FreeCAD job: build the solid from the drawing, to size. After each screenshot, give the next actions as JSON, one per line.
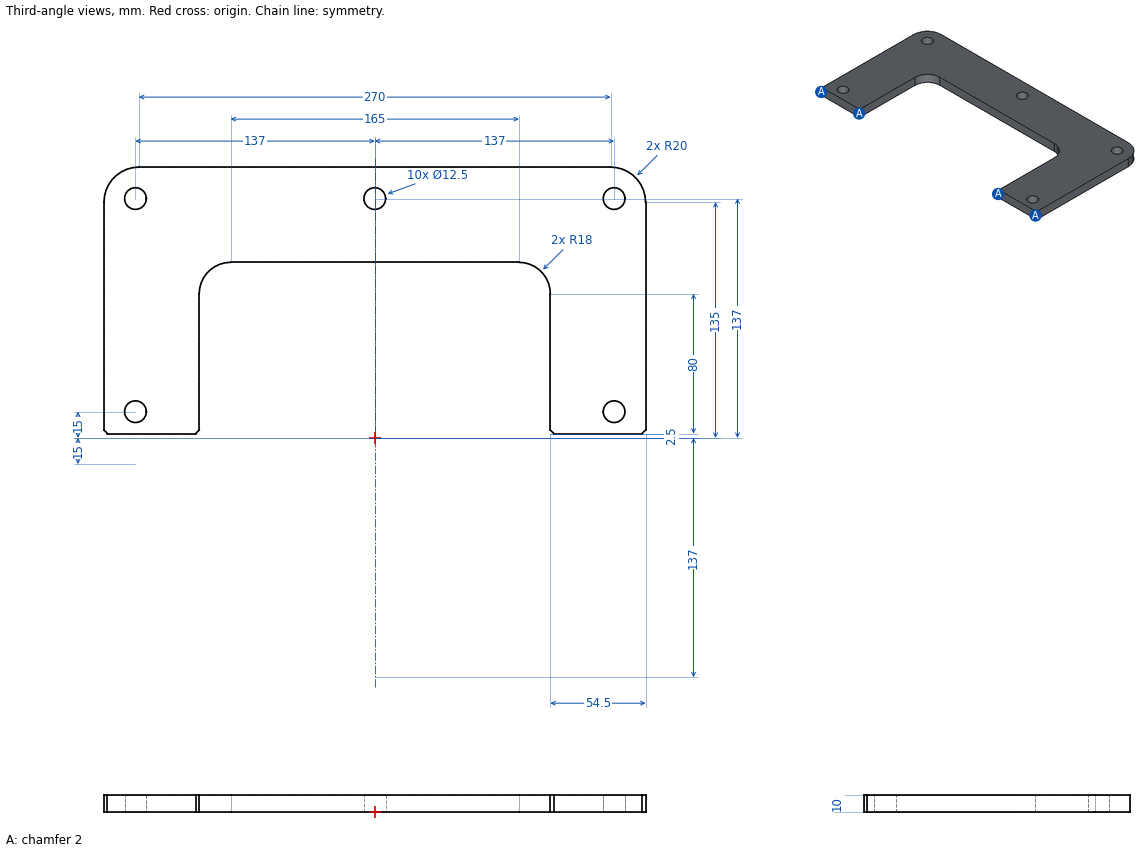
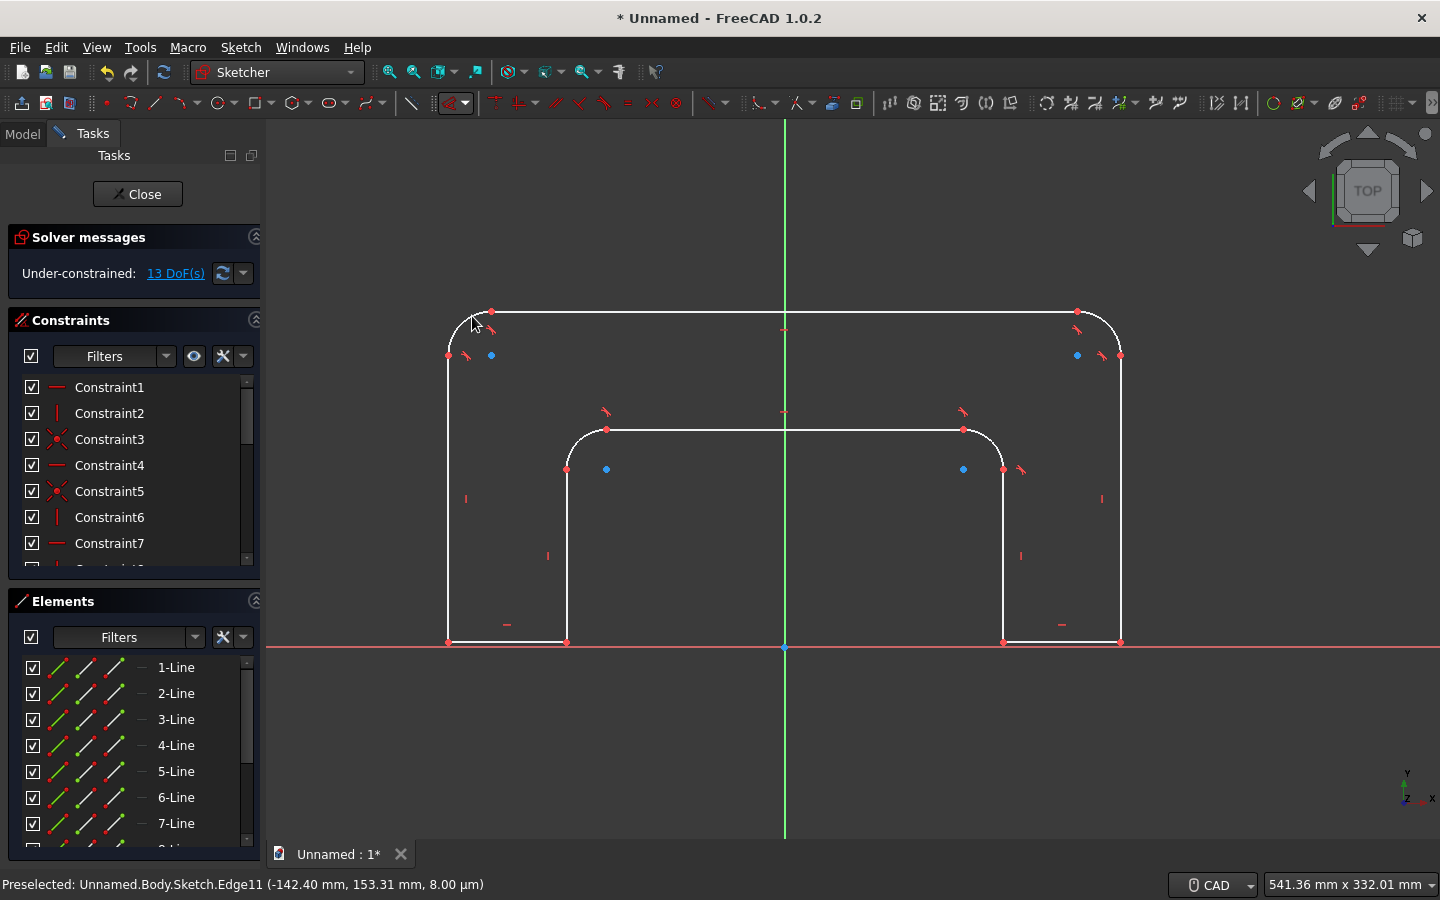
{"action": "left_click", "coordinate": [567, 590]}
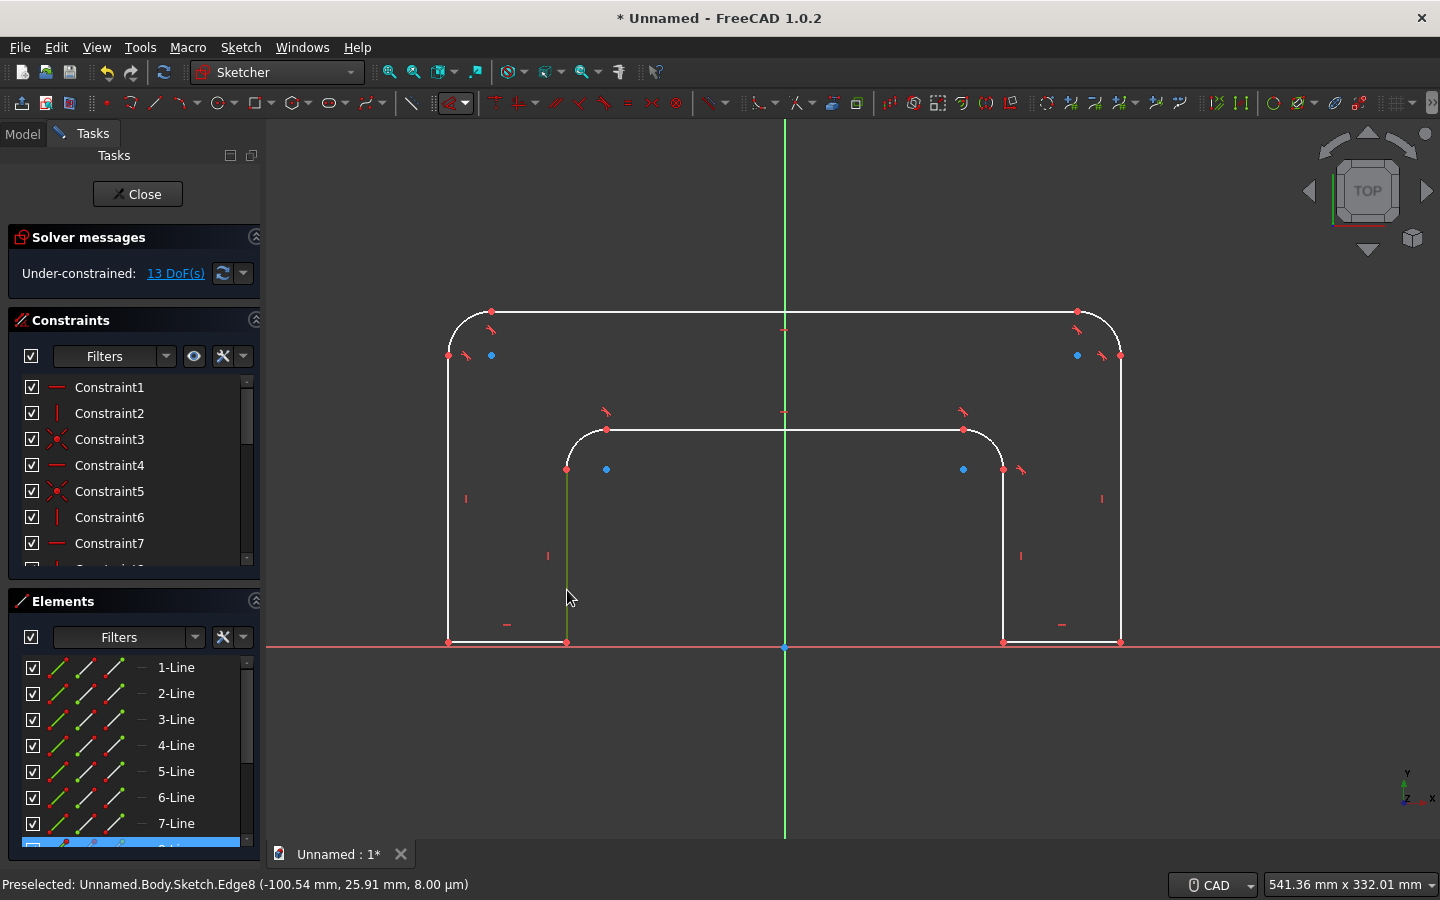
{"action": "left_click", "coordinate": [588, 434]}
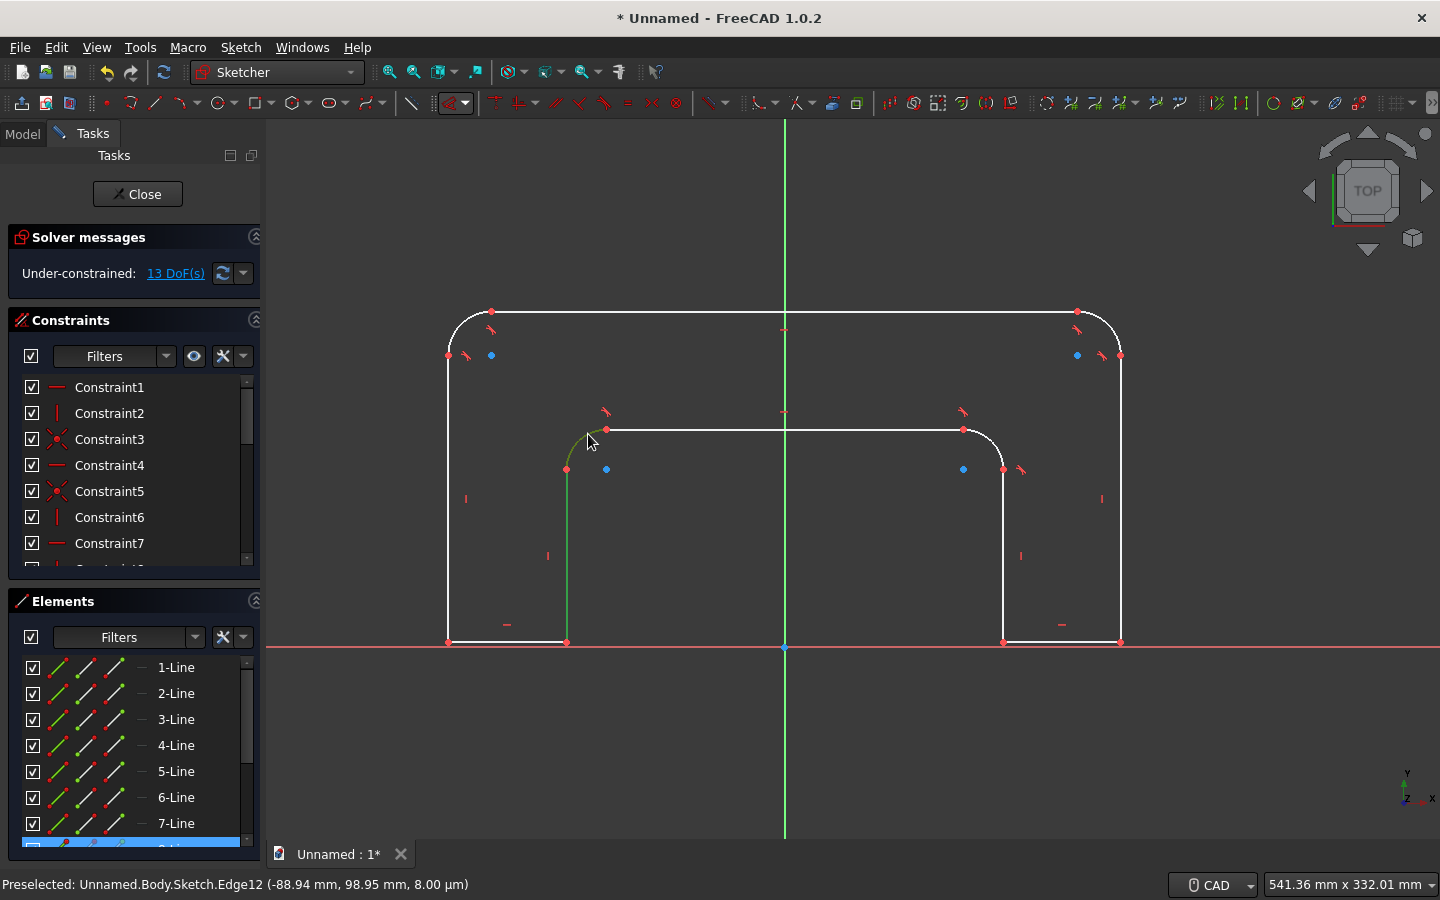
{"action": "key", "text": "t"}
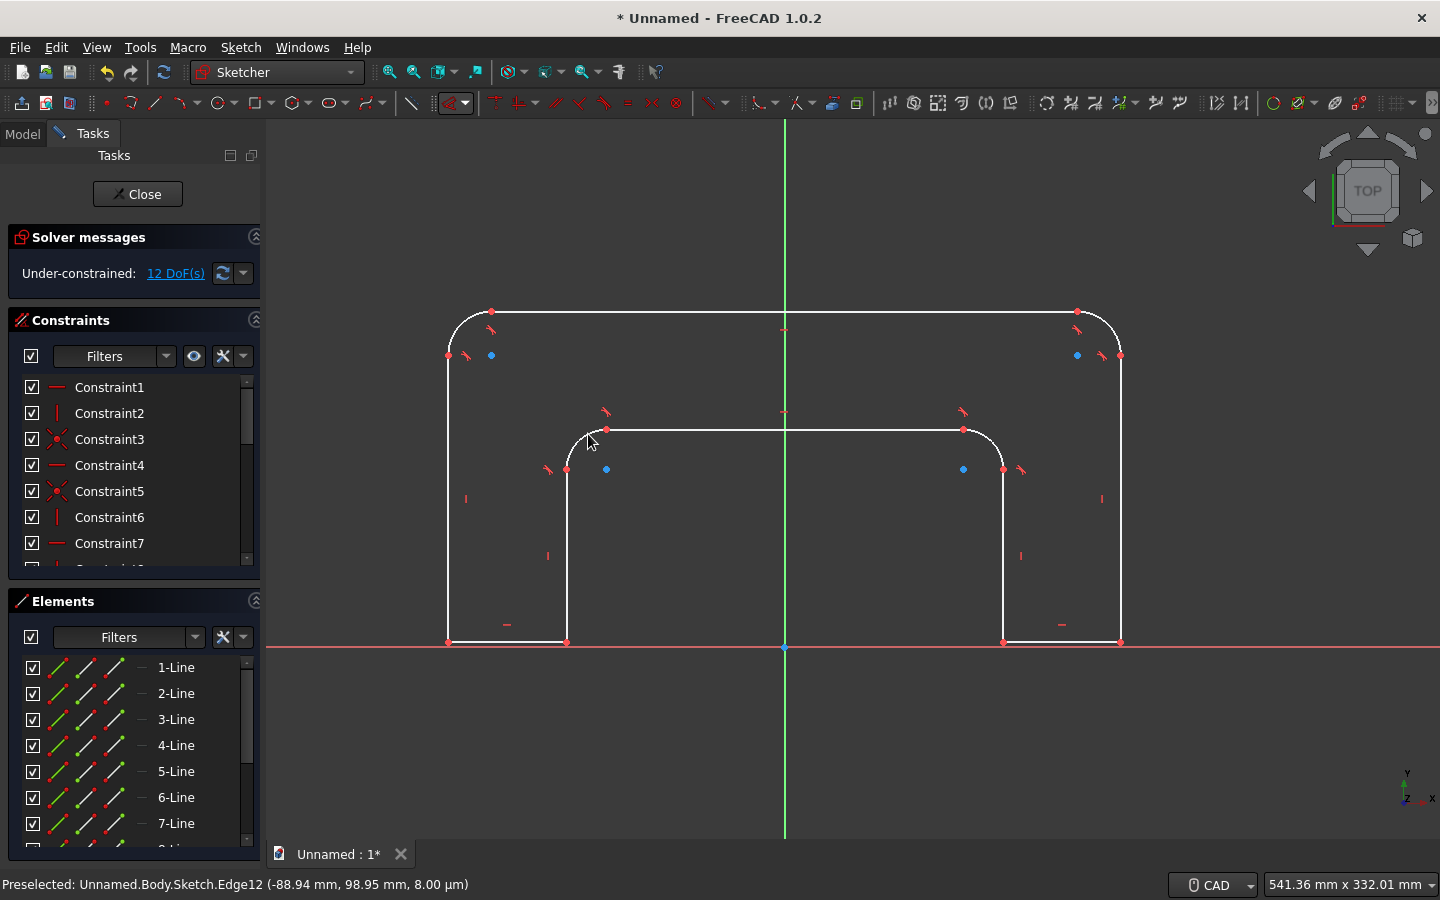
{"action": "left_click", "coordinate": [1116, 336]}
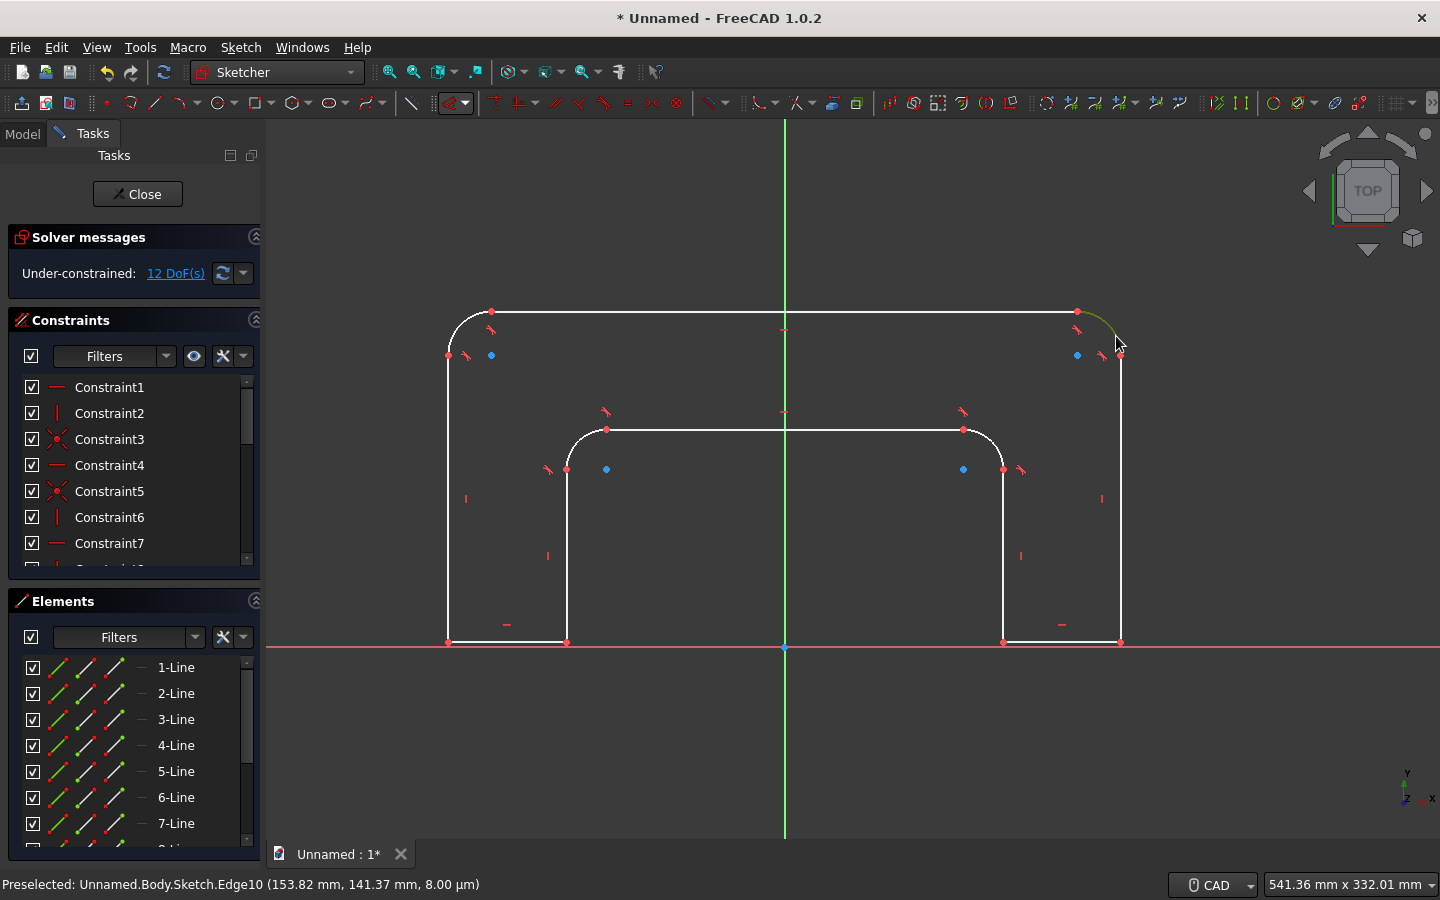
{"action": "left_click", "coordinate": [472, 316]}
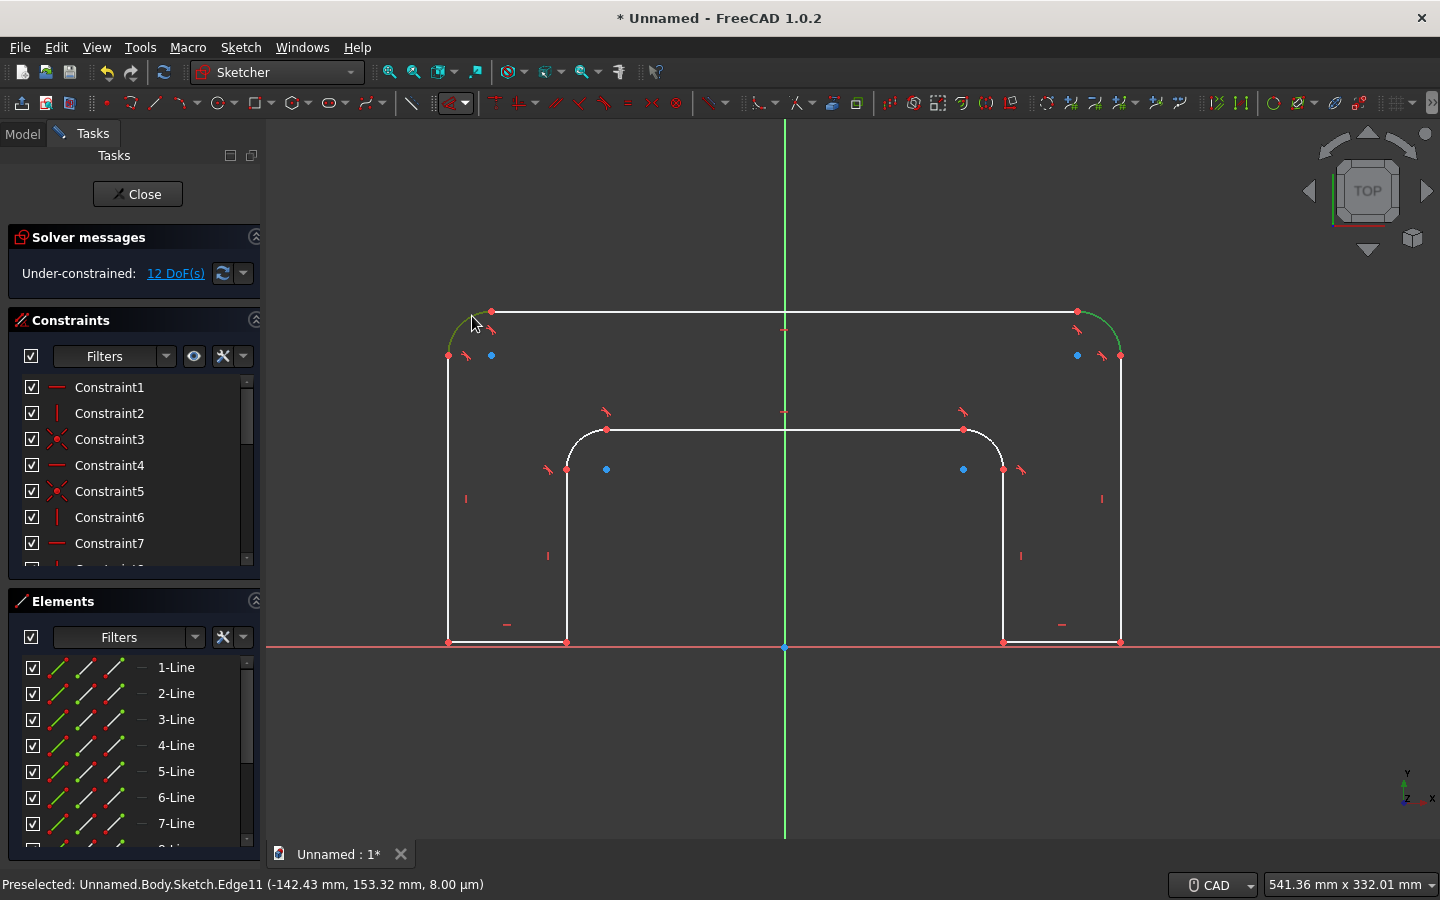
{"action": "key", "text": "e"}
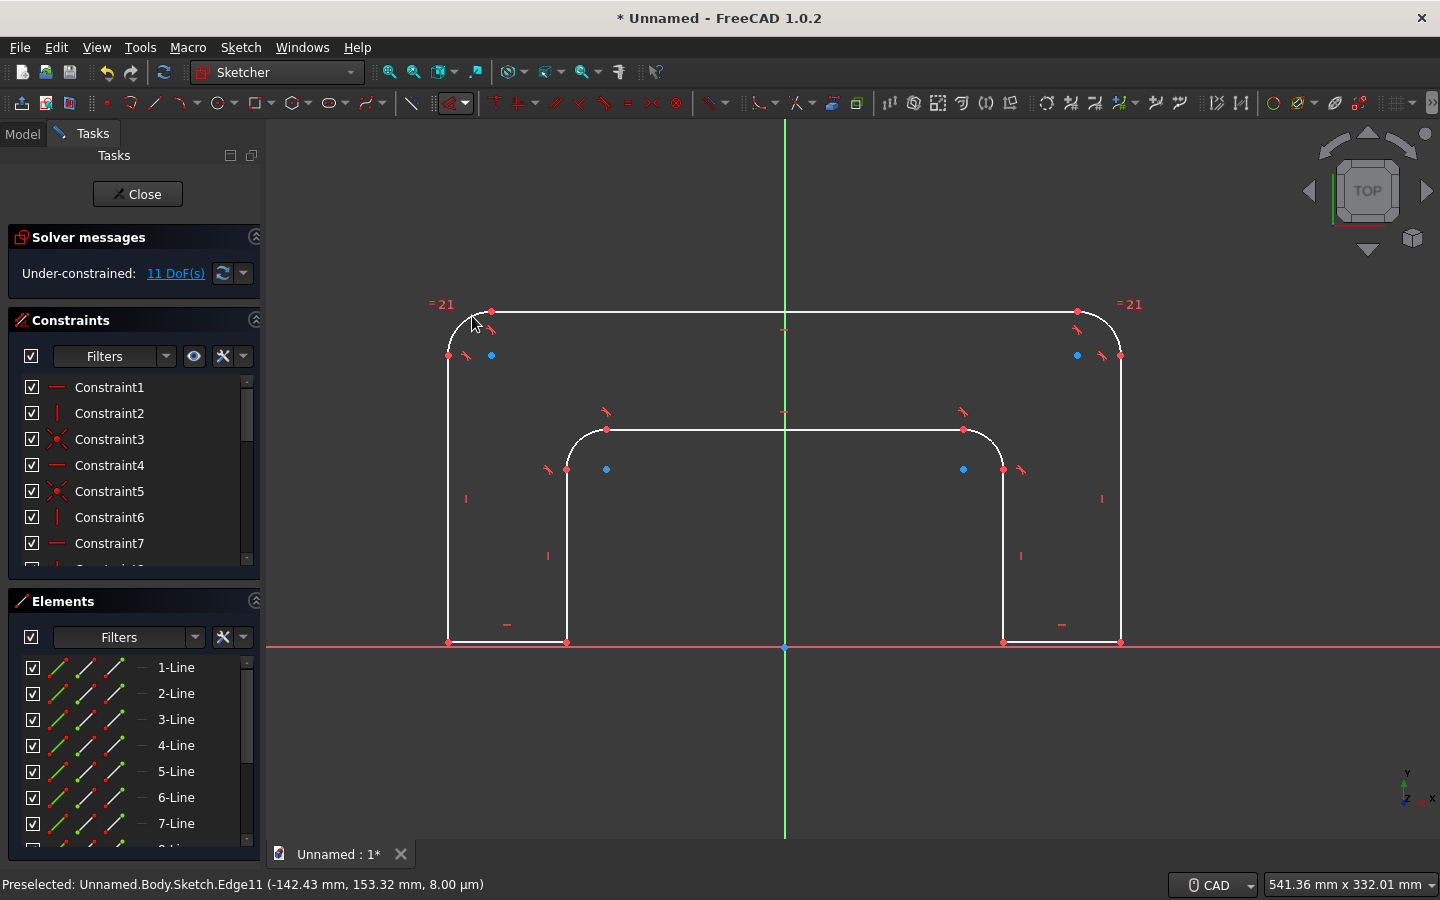
{"action": "left_click", "coordinate": [999, 452]}